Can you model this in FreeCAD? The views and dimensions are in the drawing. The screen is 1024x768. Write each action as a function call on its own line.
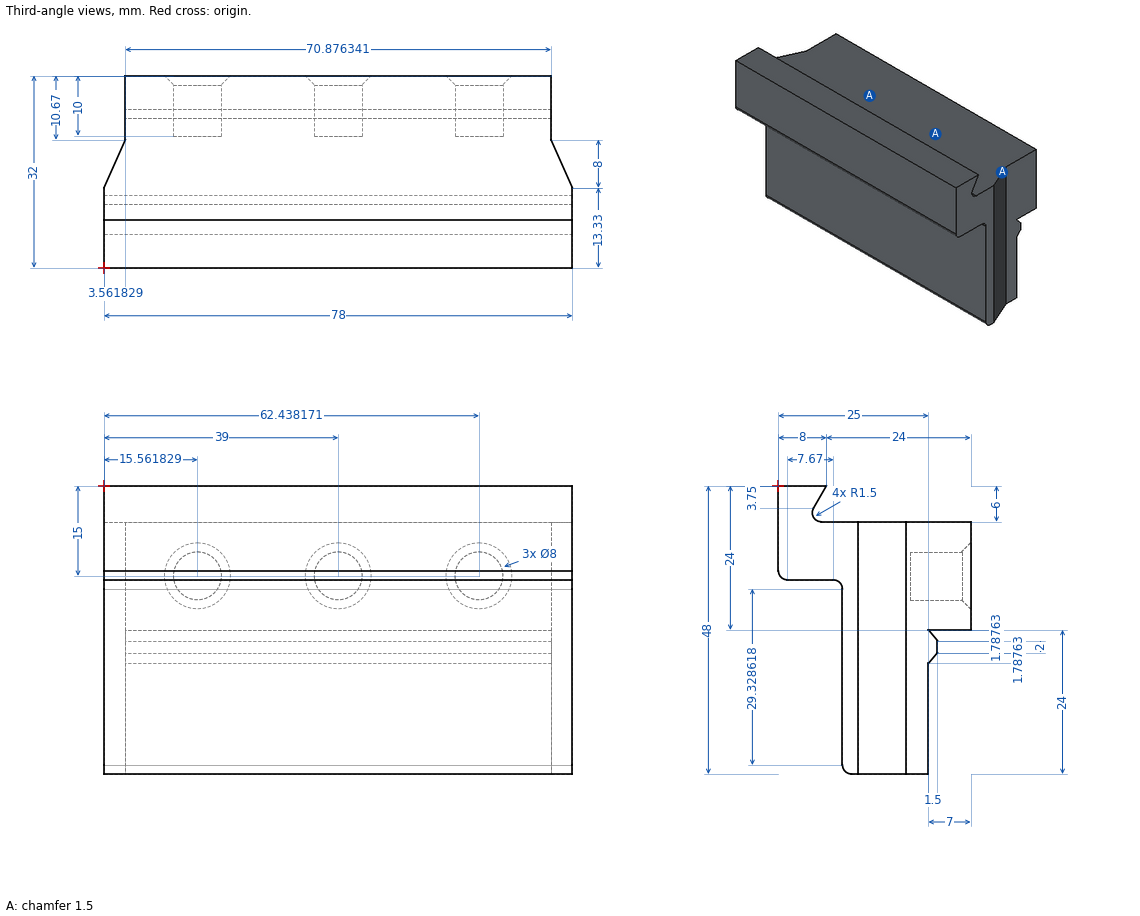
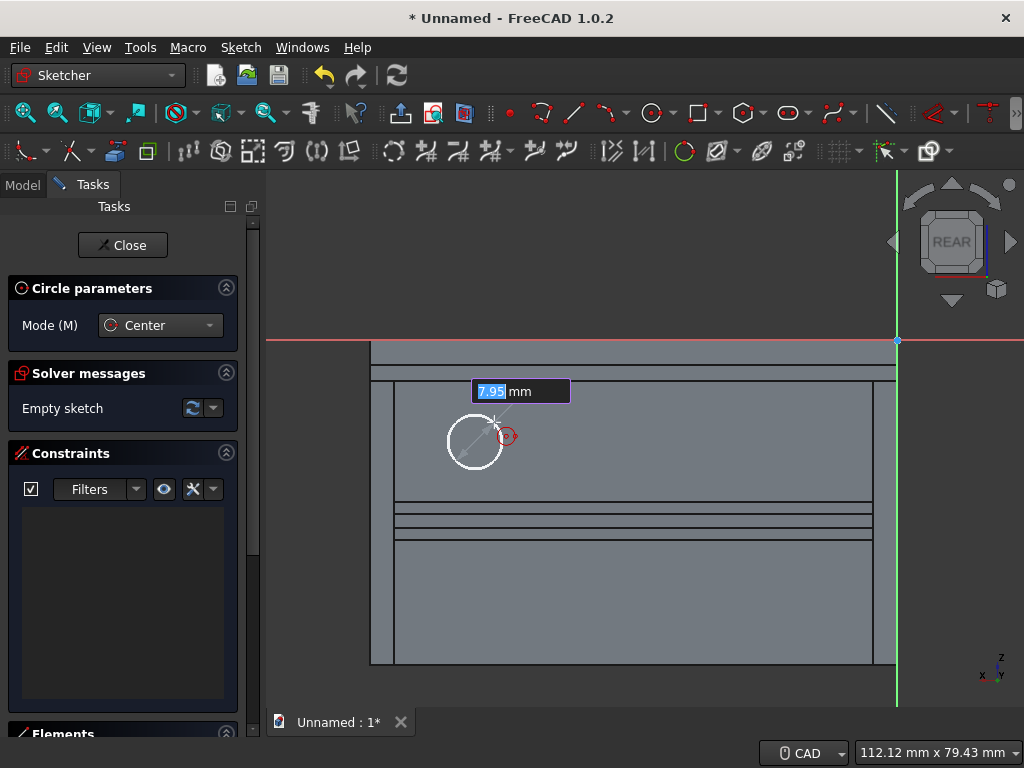
text(8)
key(Return)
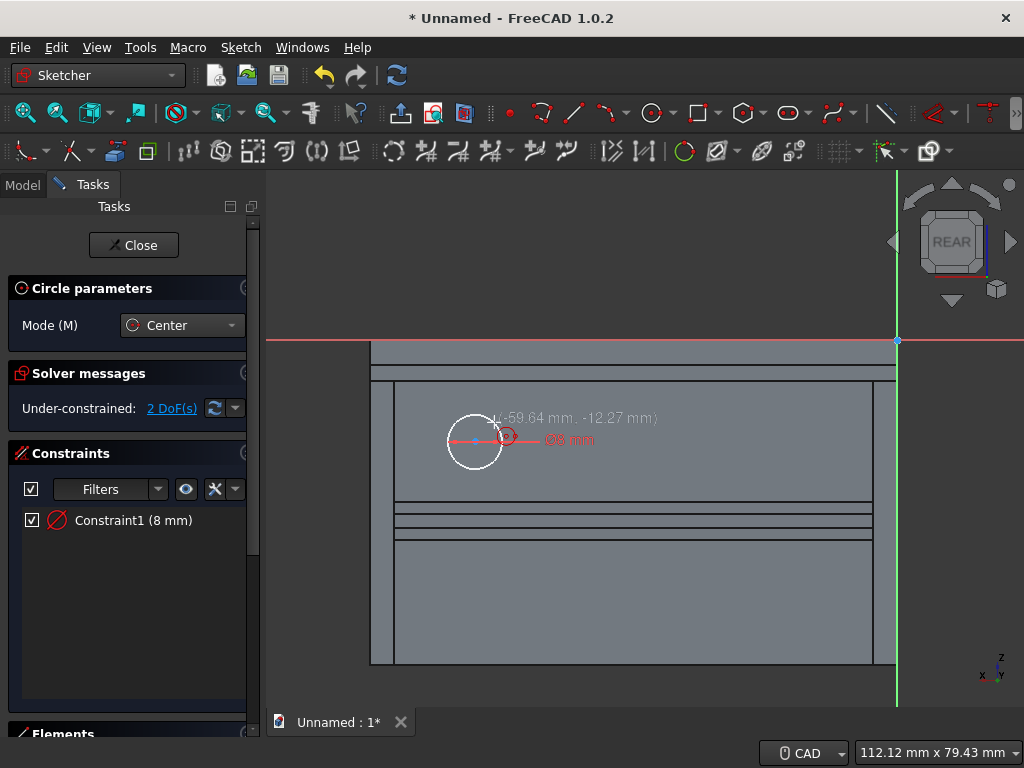
click(634, 441)
move(653, 422)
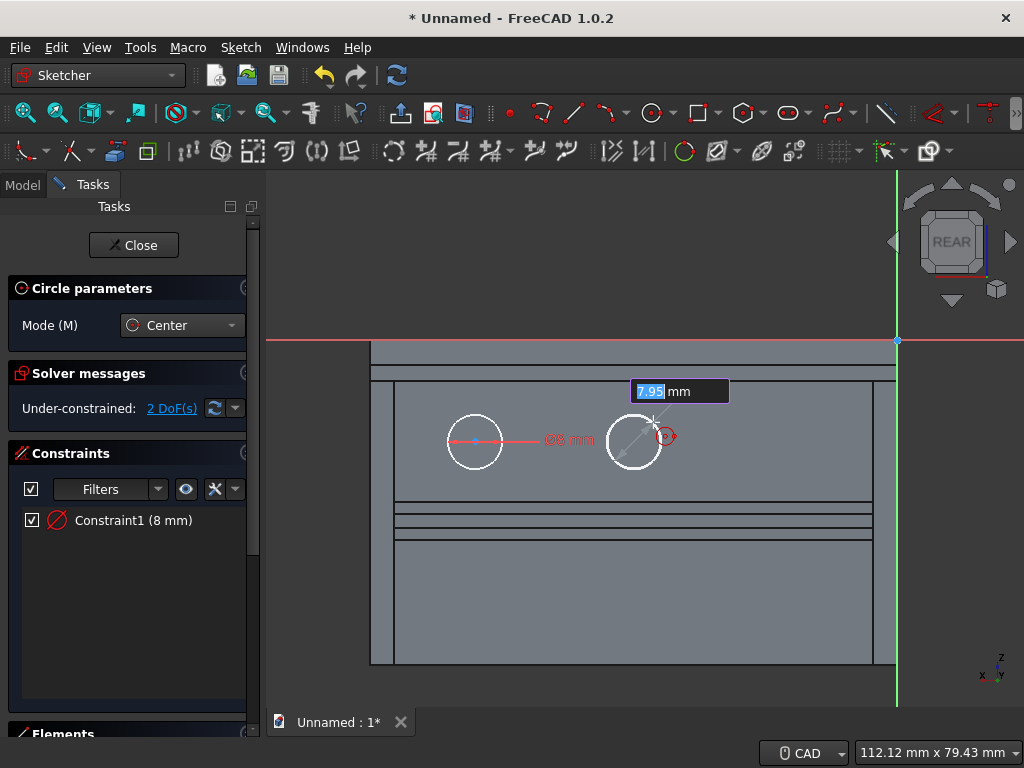
text(8)
key(Return)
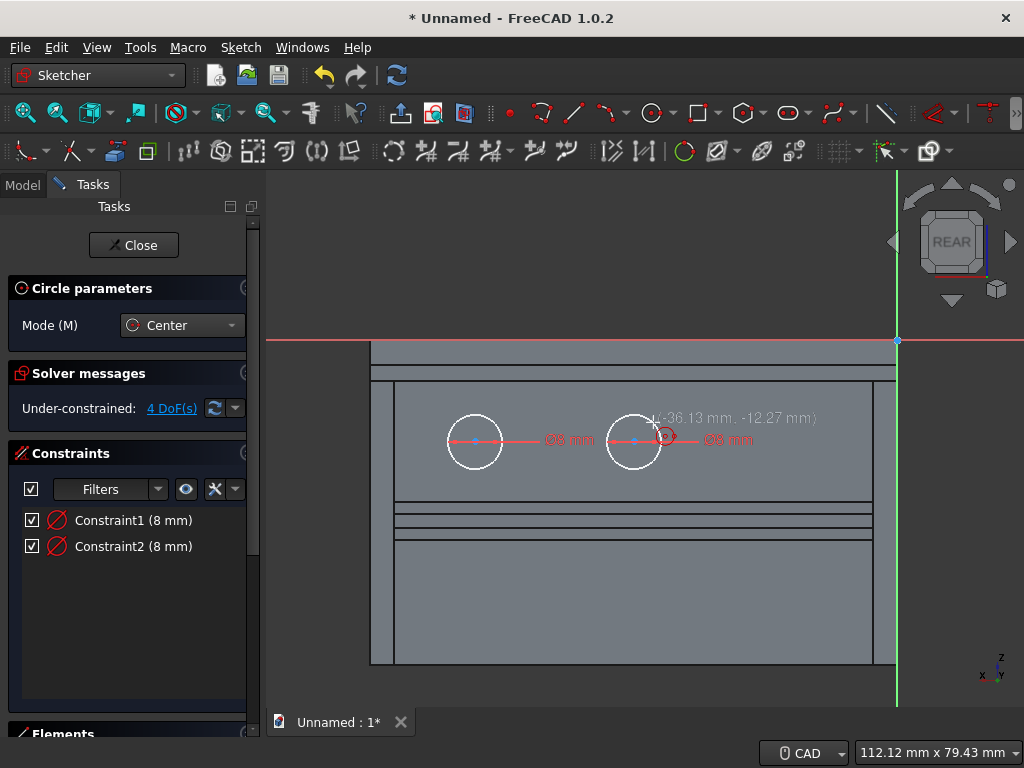
click(792, 441)
move(811, 422)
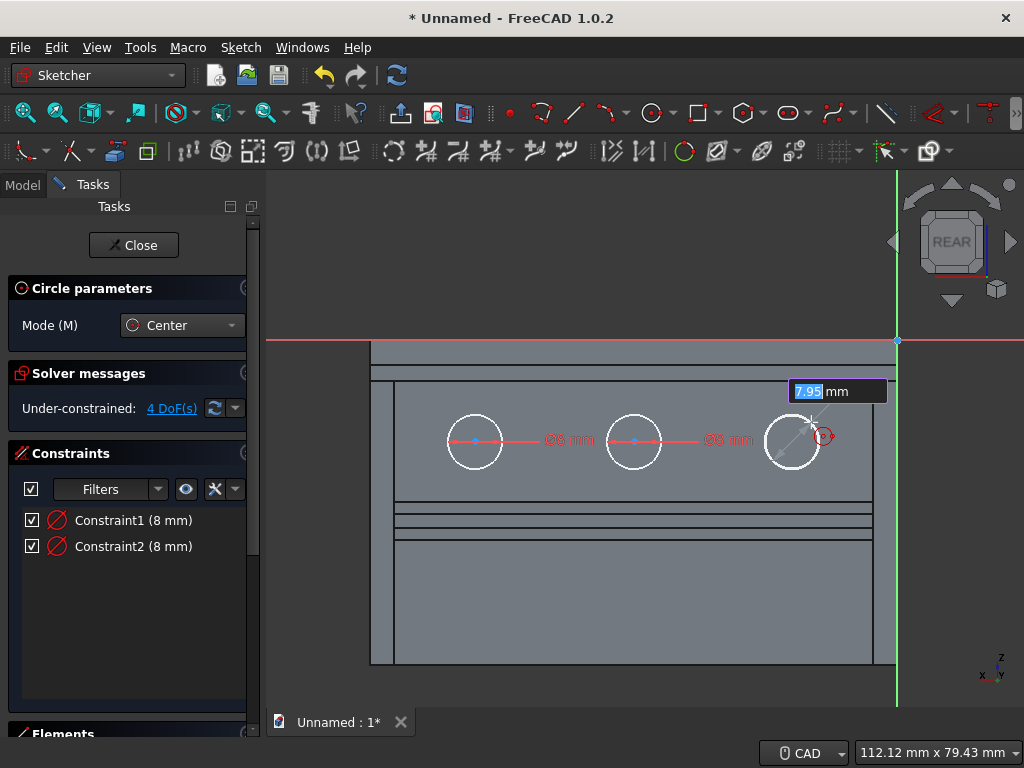
text(8)
key(Return)
key(Escape)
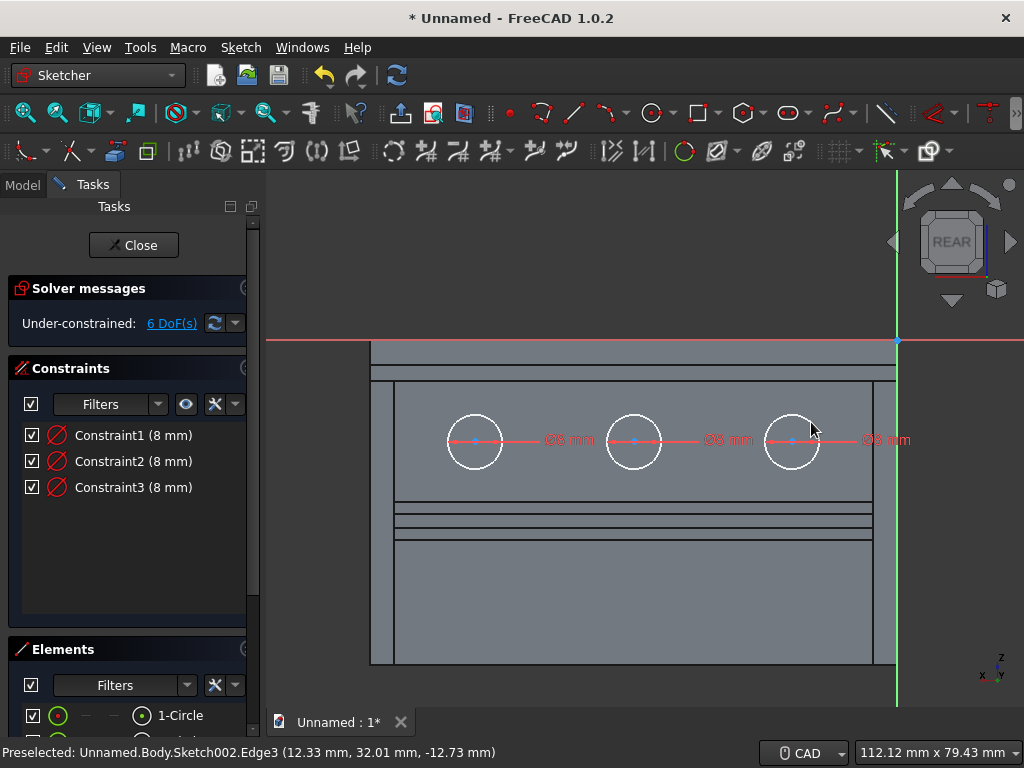
click(934, 114)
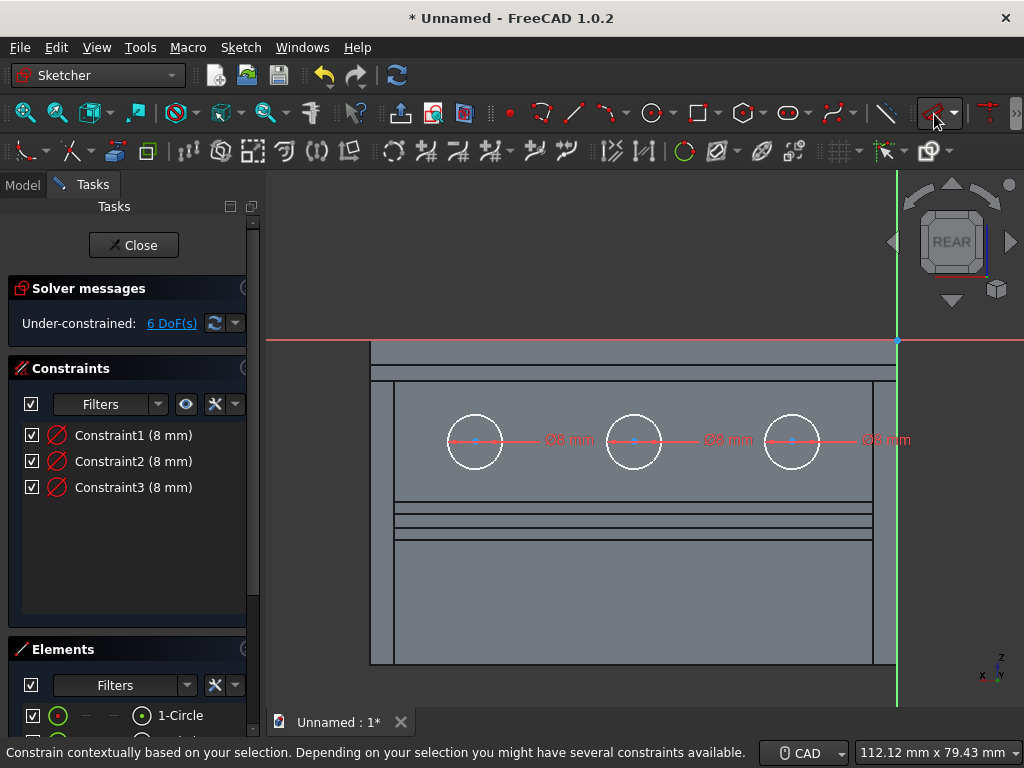
click(475, 442)
click(441, 391)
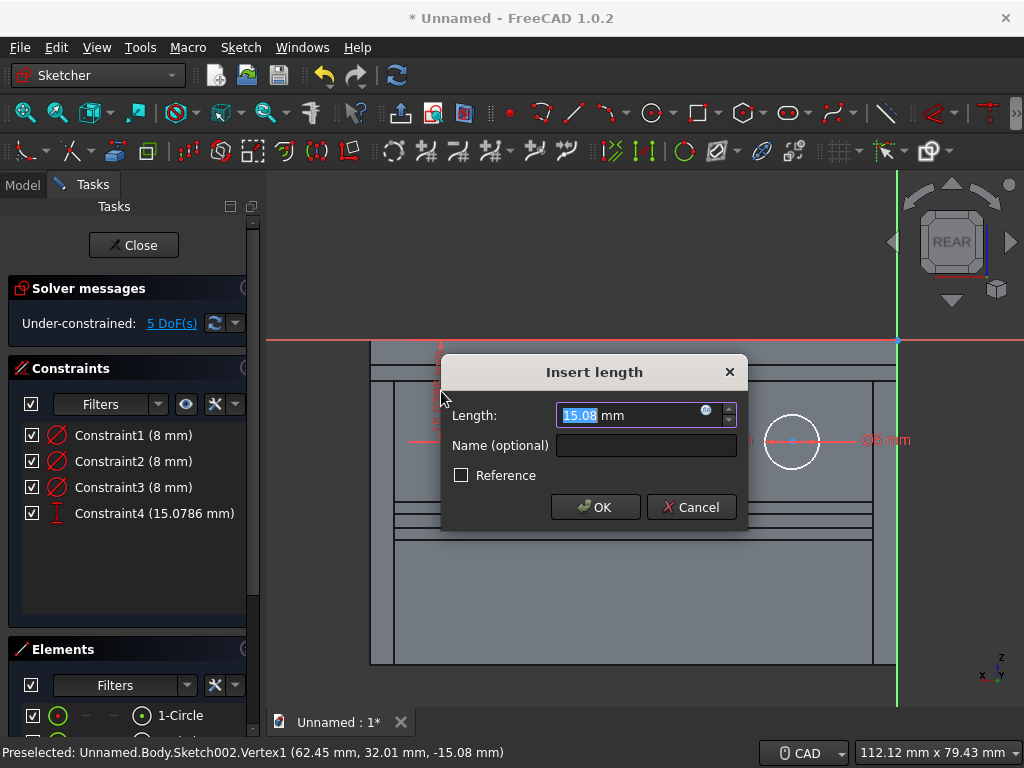
text(15)
key(Return)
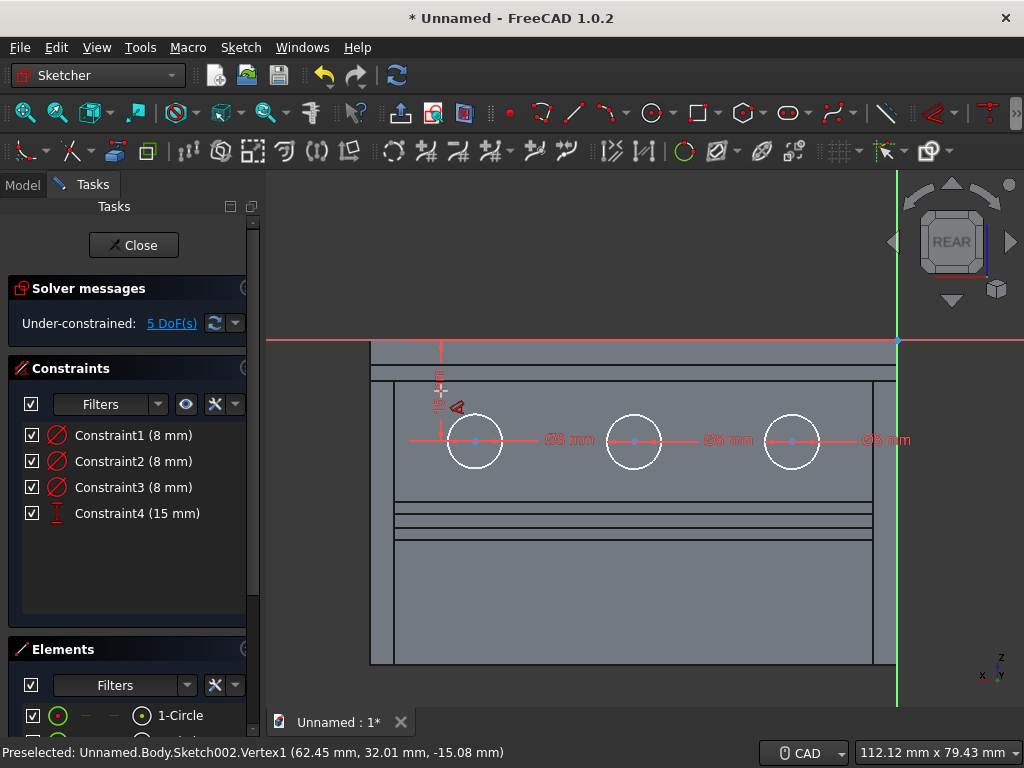
click(634, 442)
click(747, 306)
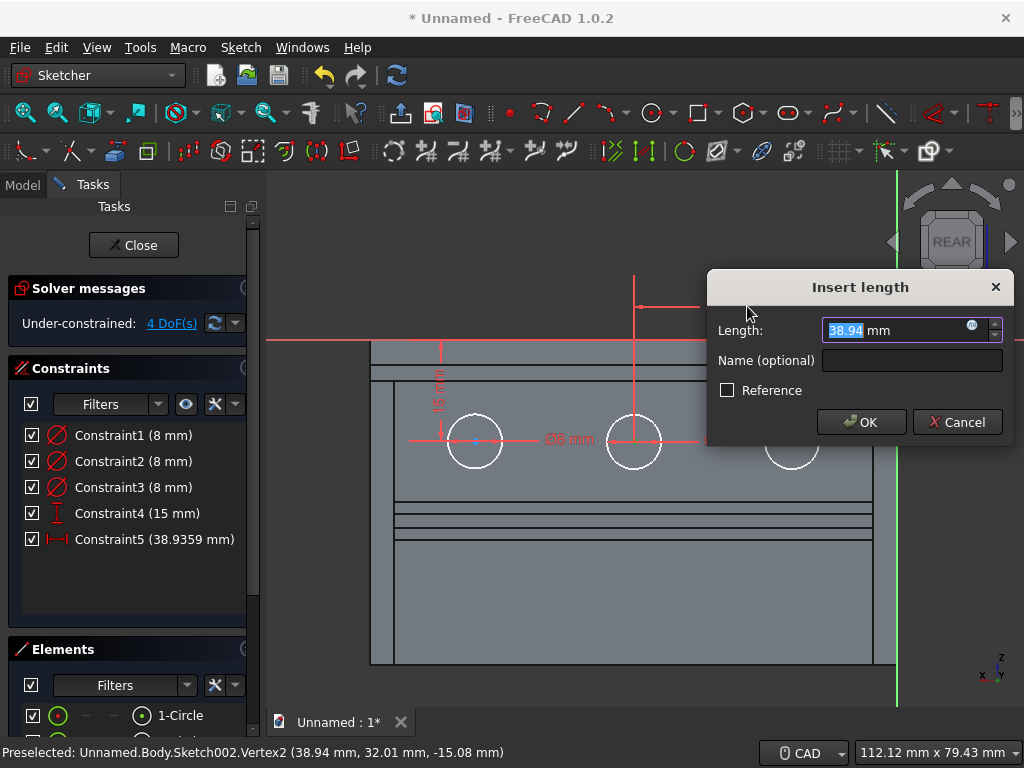
text(39)
key(Return)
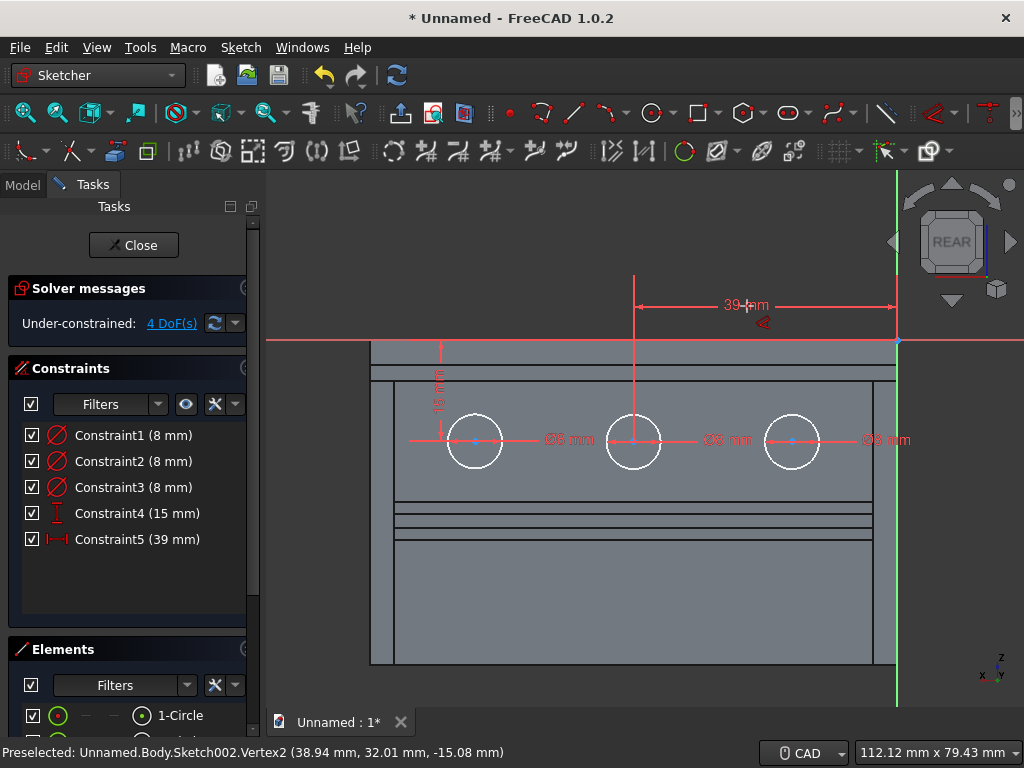
click(634, 442)
click(600, 391)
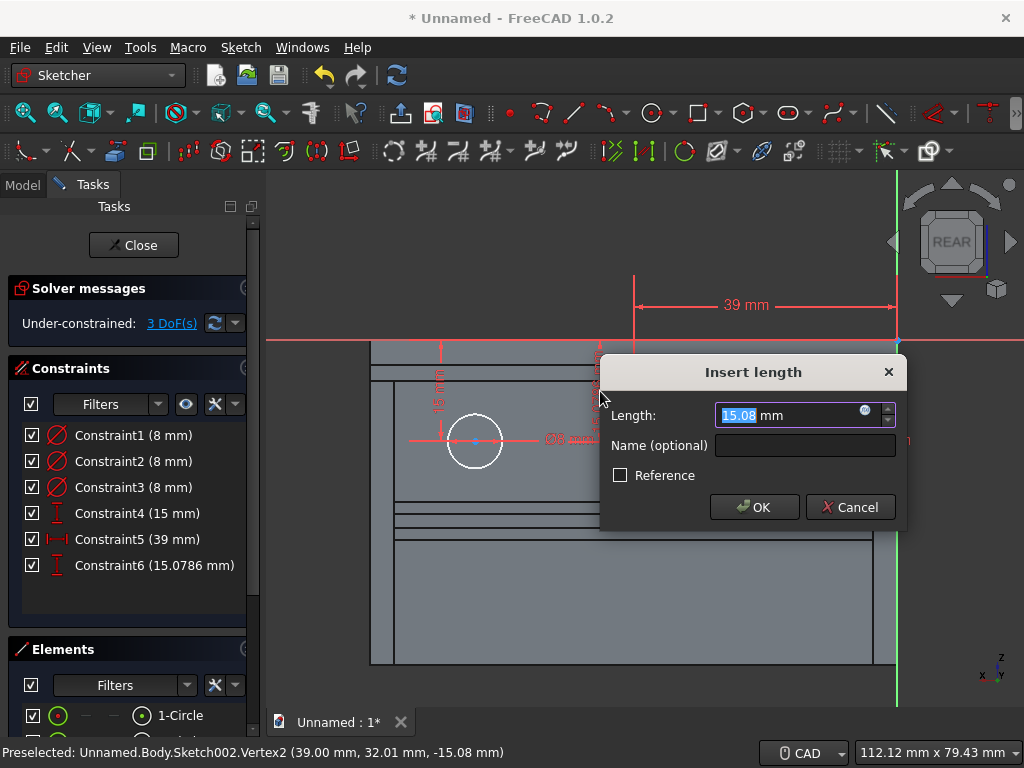
text(15)
key(Return)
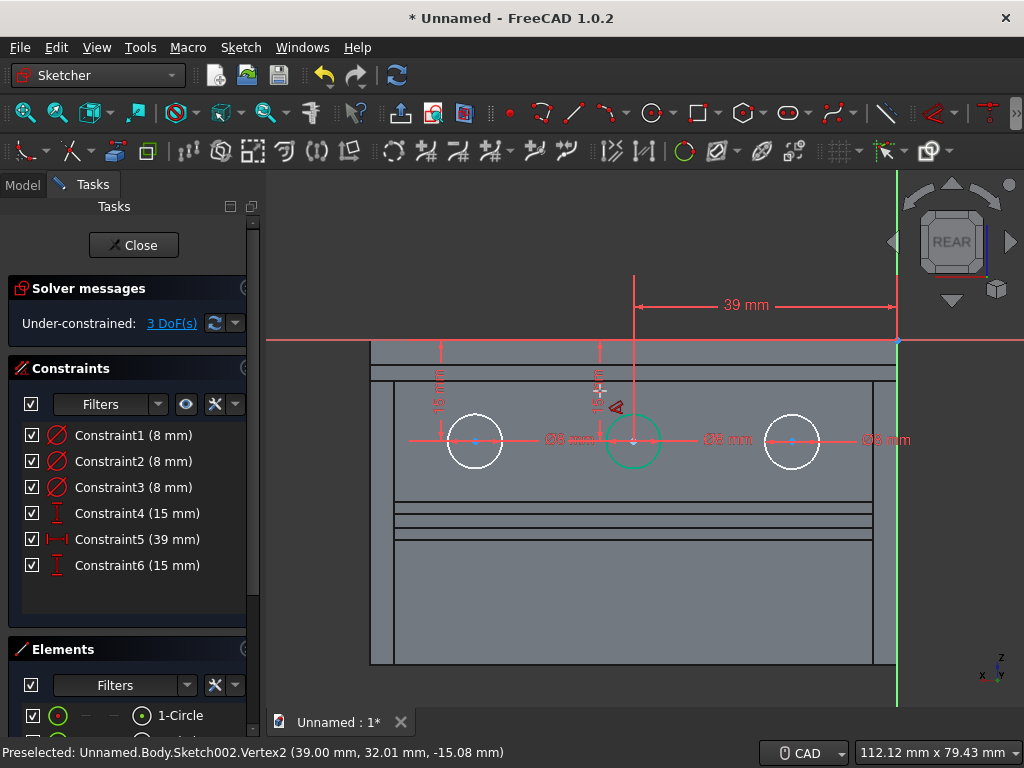
click(792, 442)
click(758, 391)